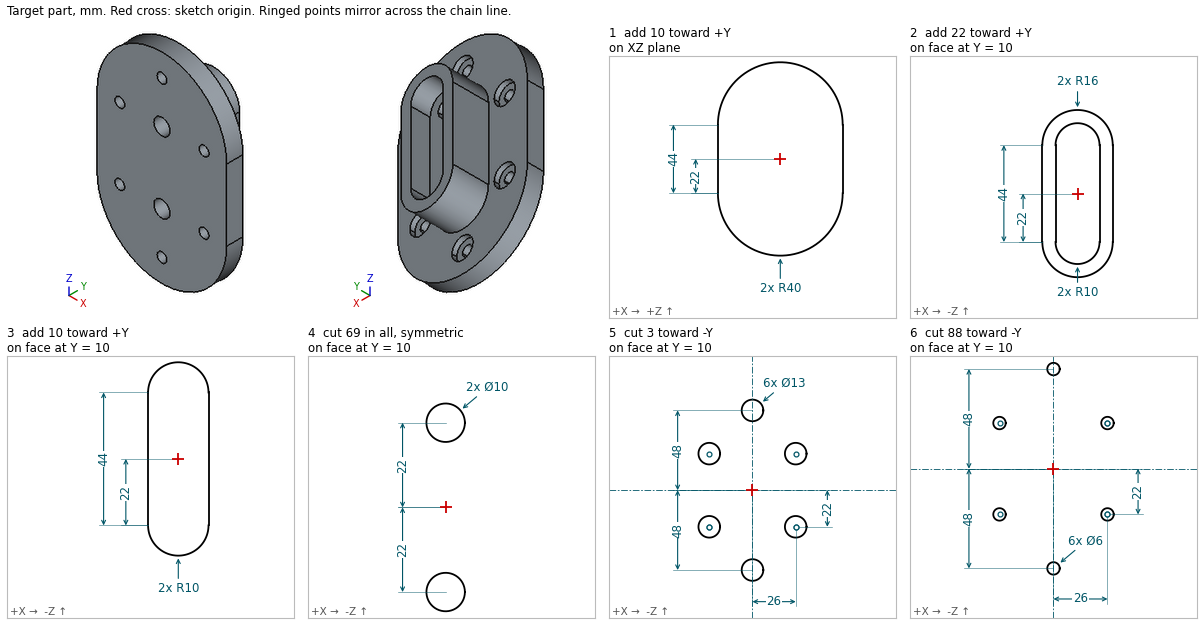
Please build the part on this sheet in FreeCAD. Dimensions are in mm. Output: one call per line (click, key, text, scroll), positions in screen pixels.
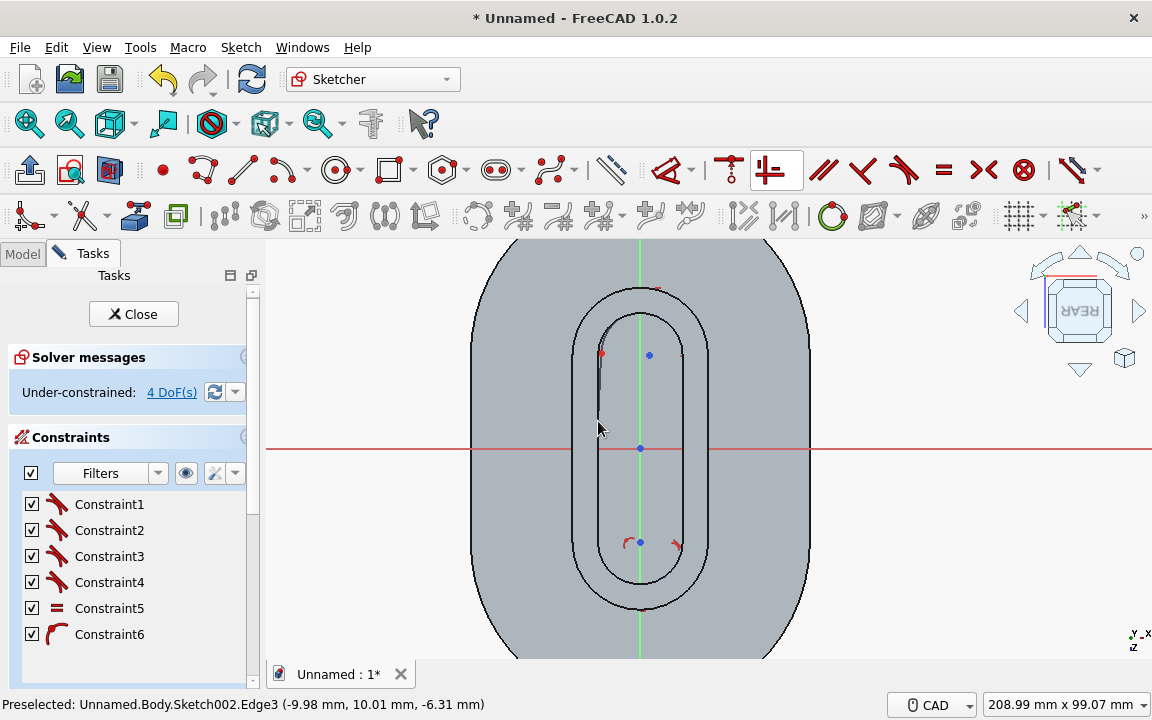
click(595, 485)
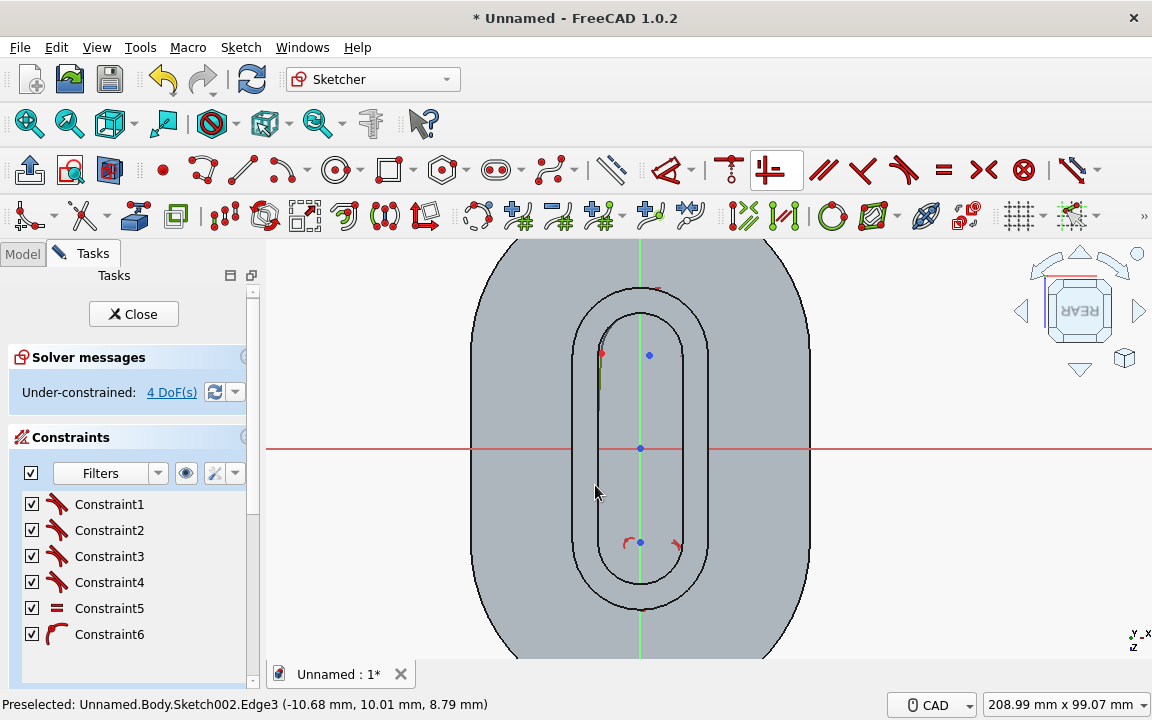
click(798, 170)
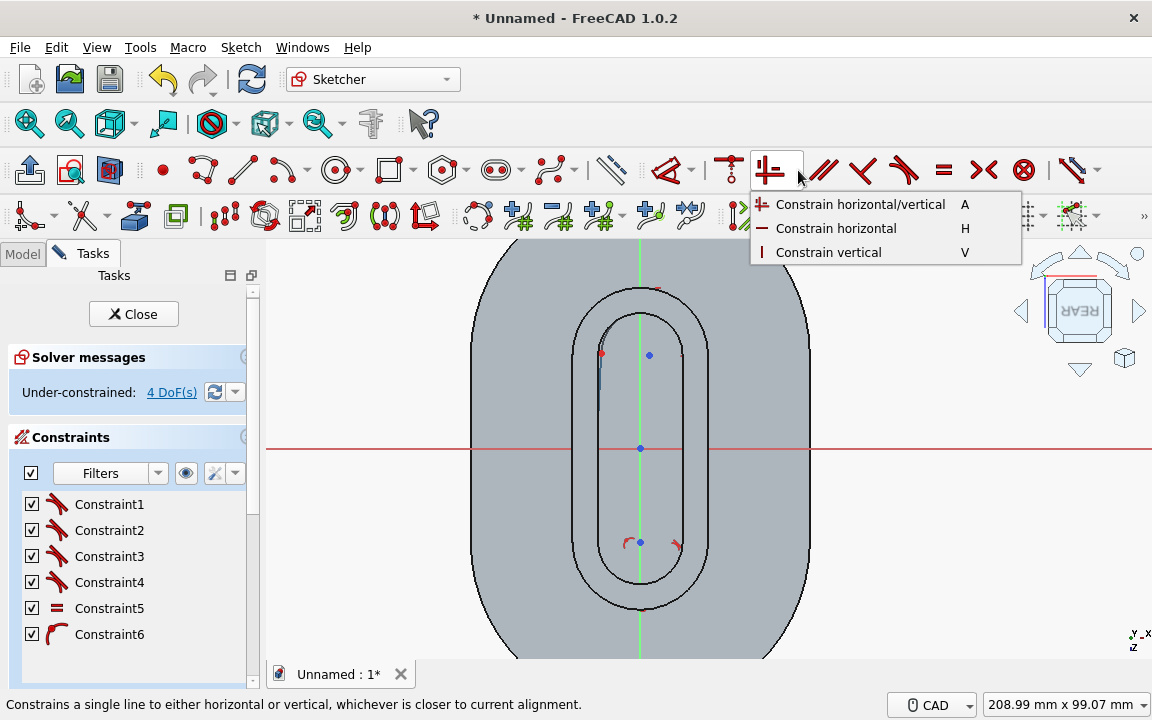
click(886, 252)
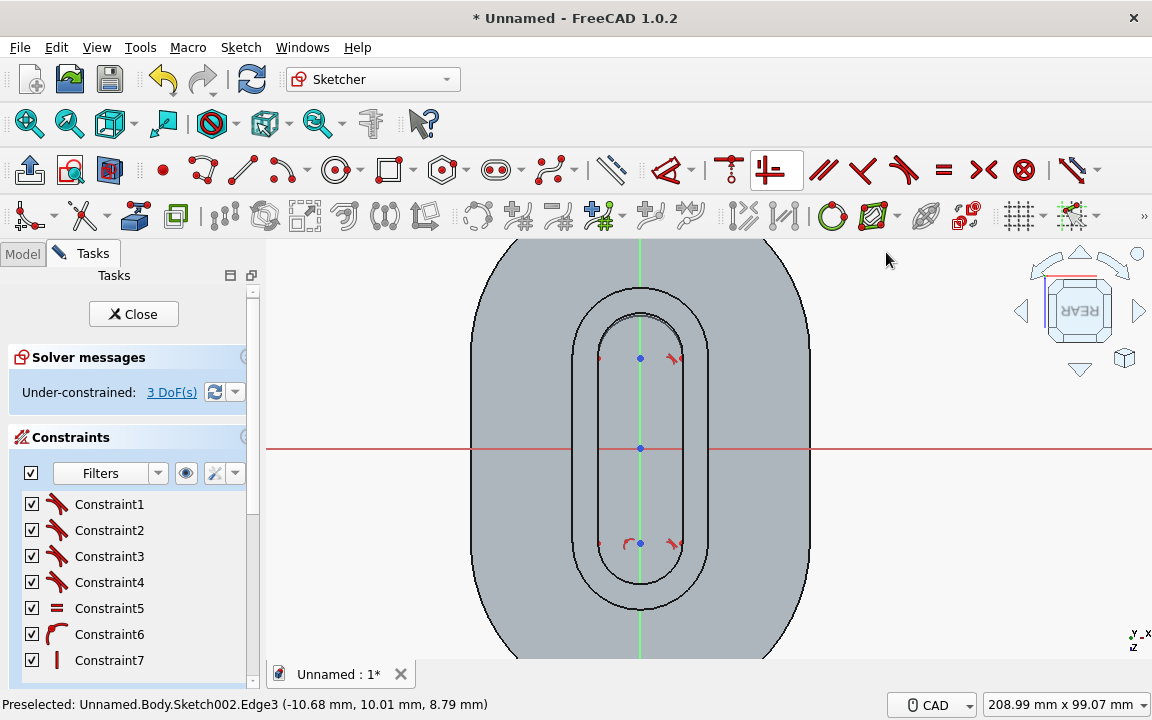
click(666, 170)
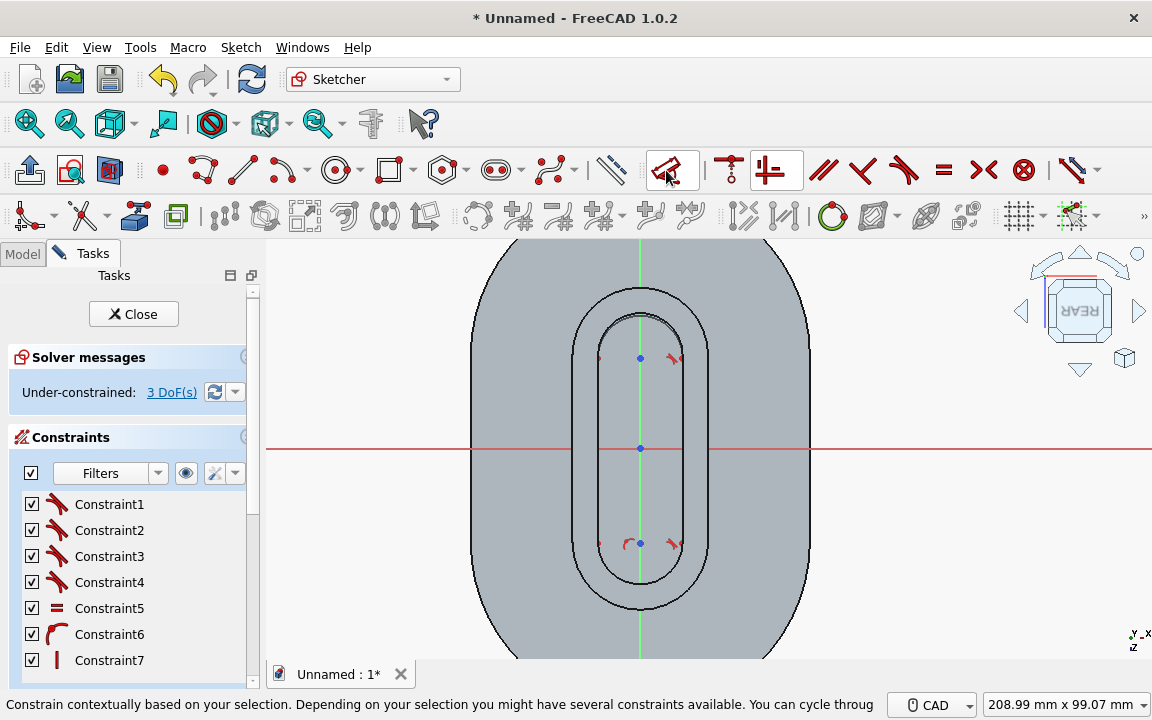
click(615, 577)
click(596, 603)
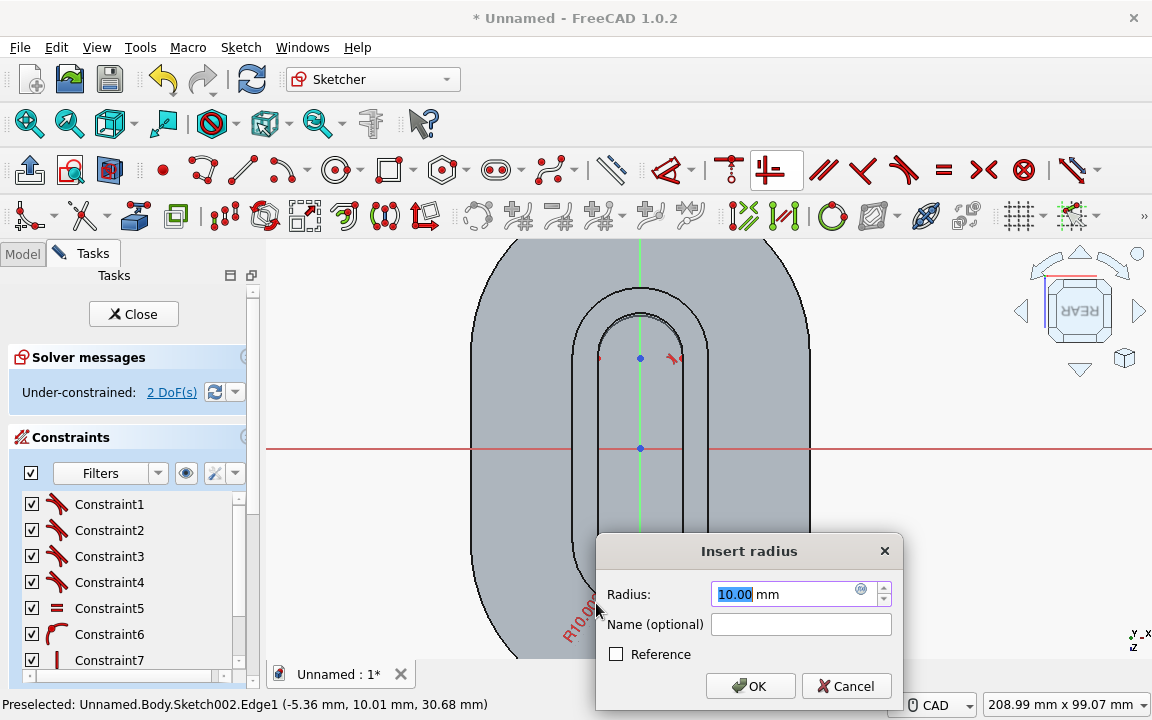
text(10)
key(Return)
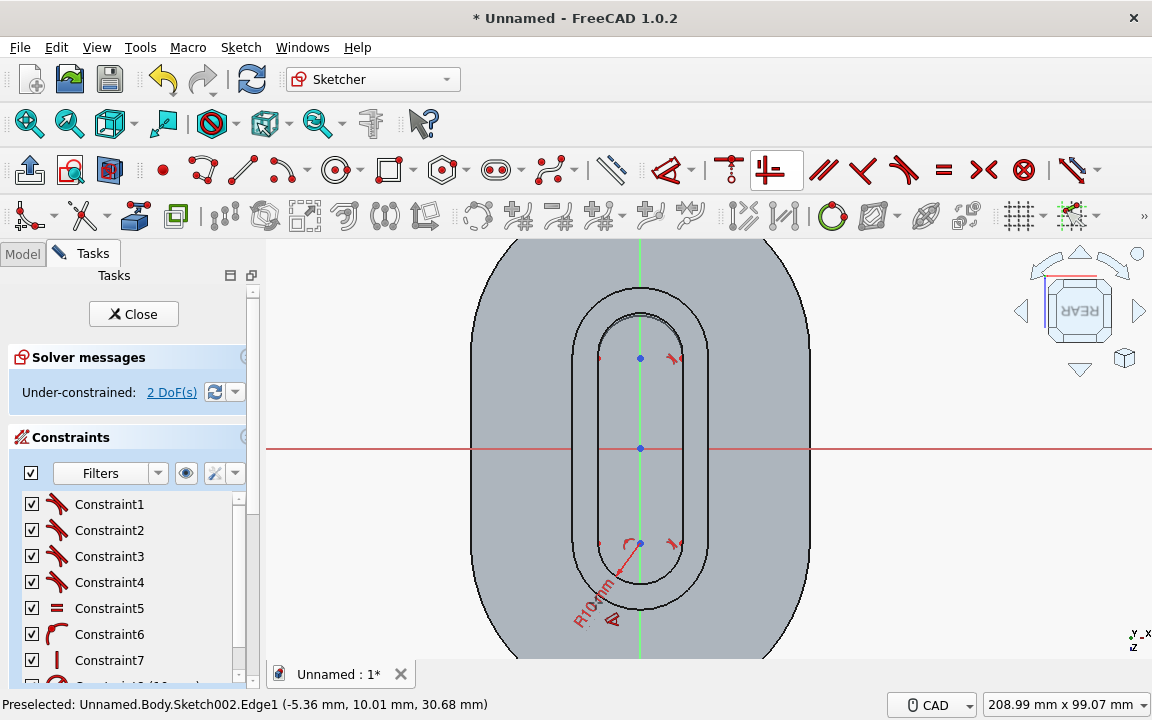
click(598, 488)
click(564, 408)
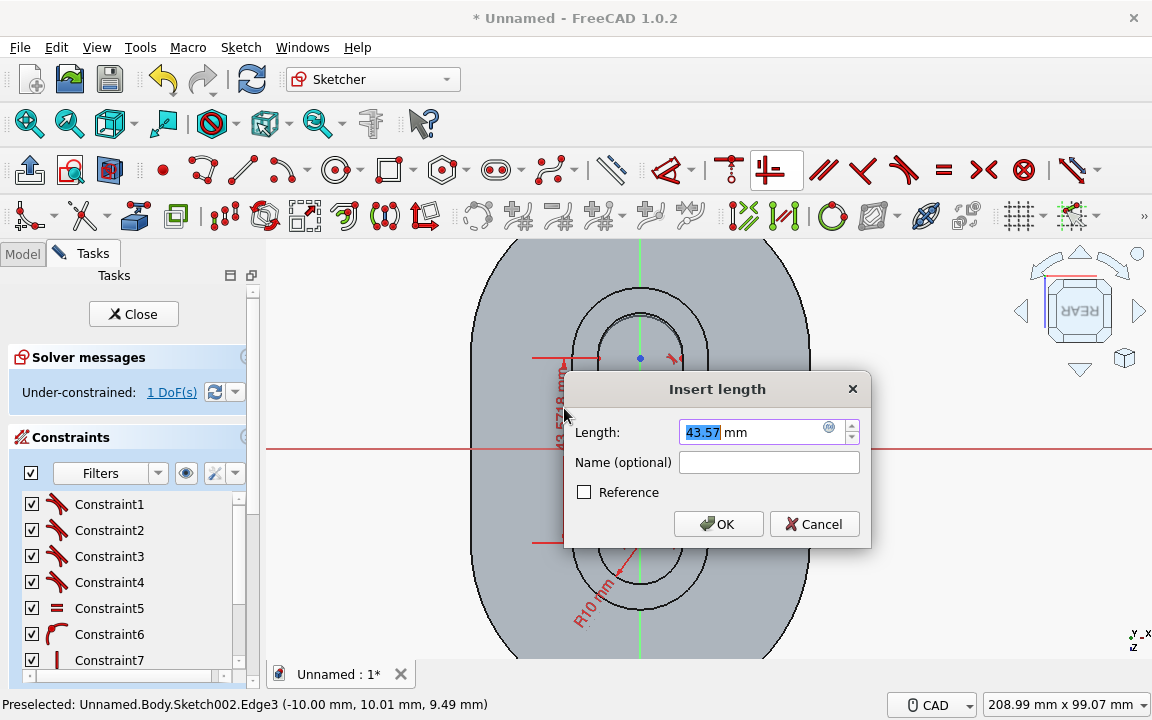
text(44)
key(Return)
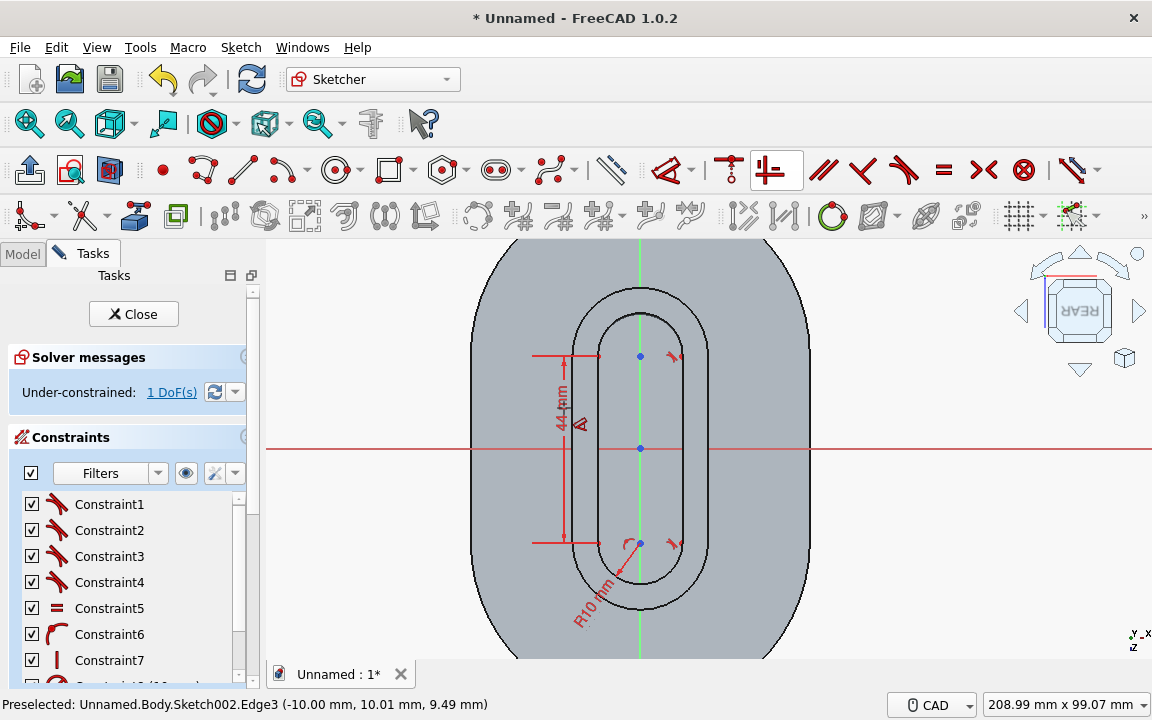
click(598, 543)
click(564, 496)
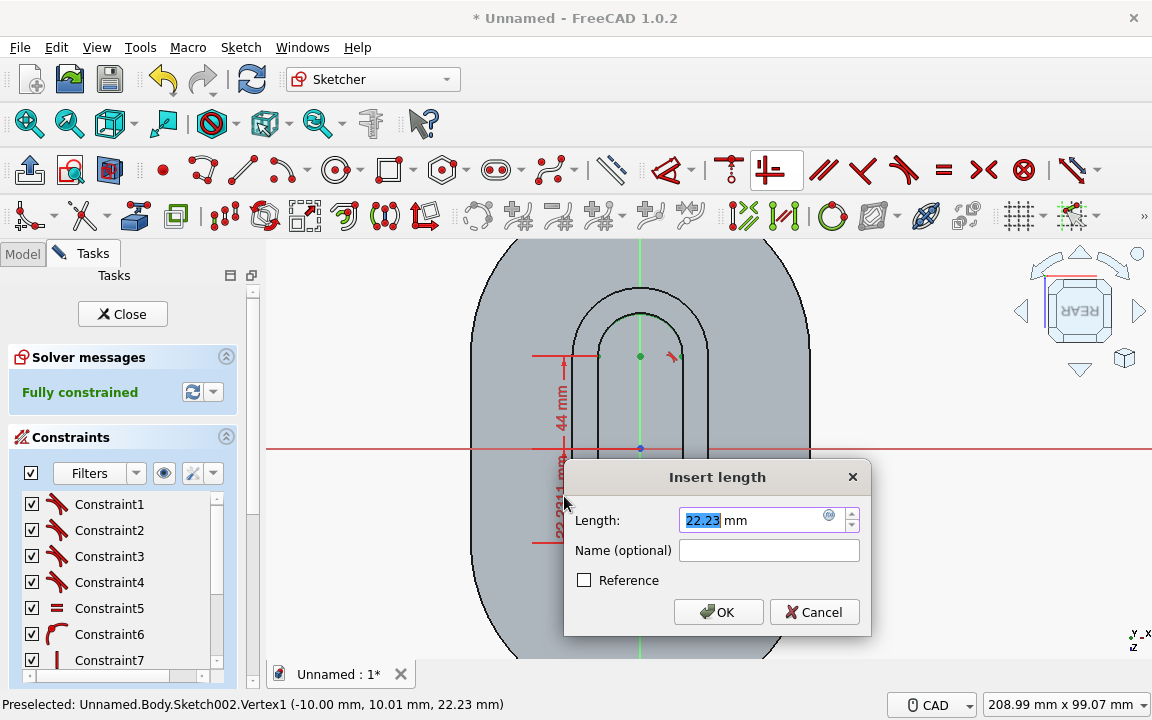
text(22)
key(Return)
key(Escape)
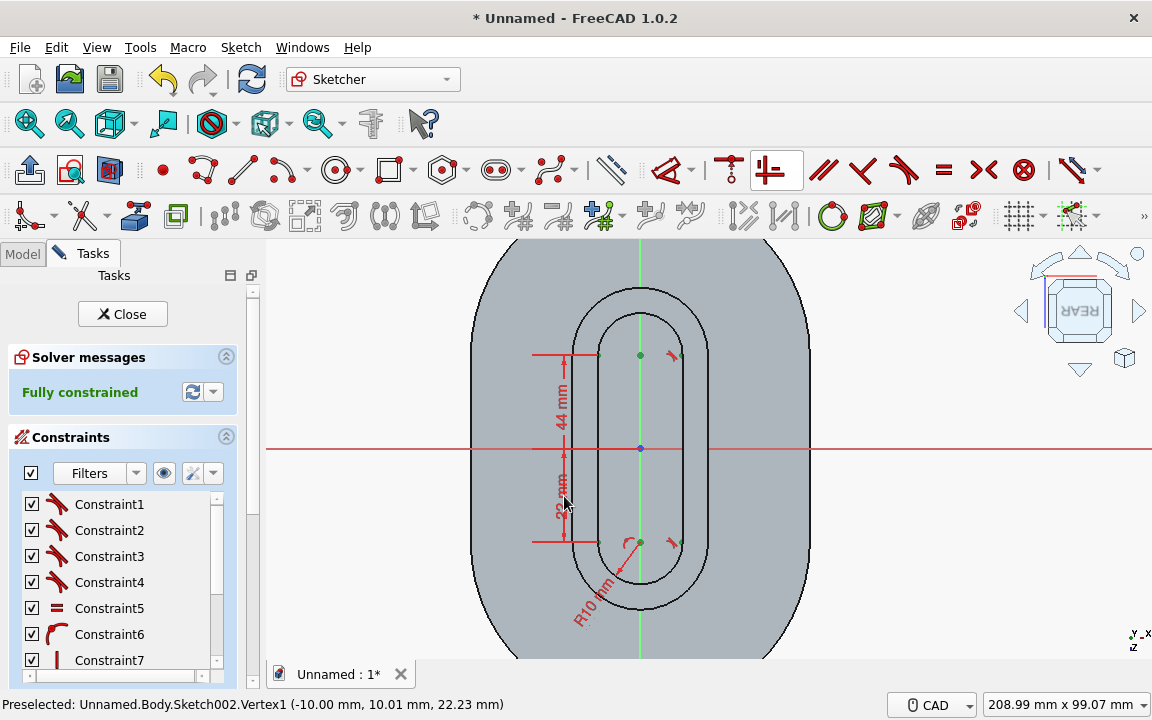
click(123, 314)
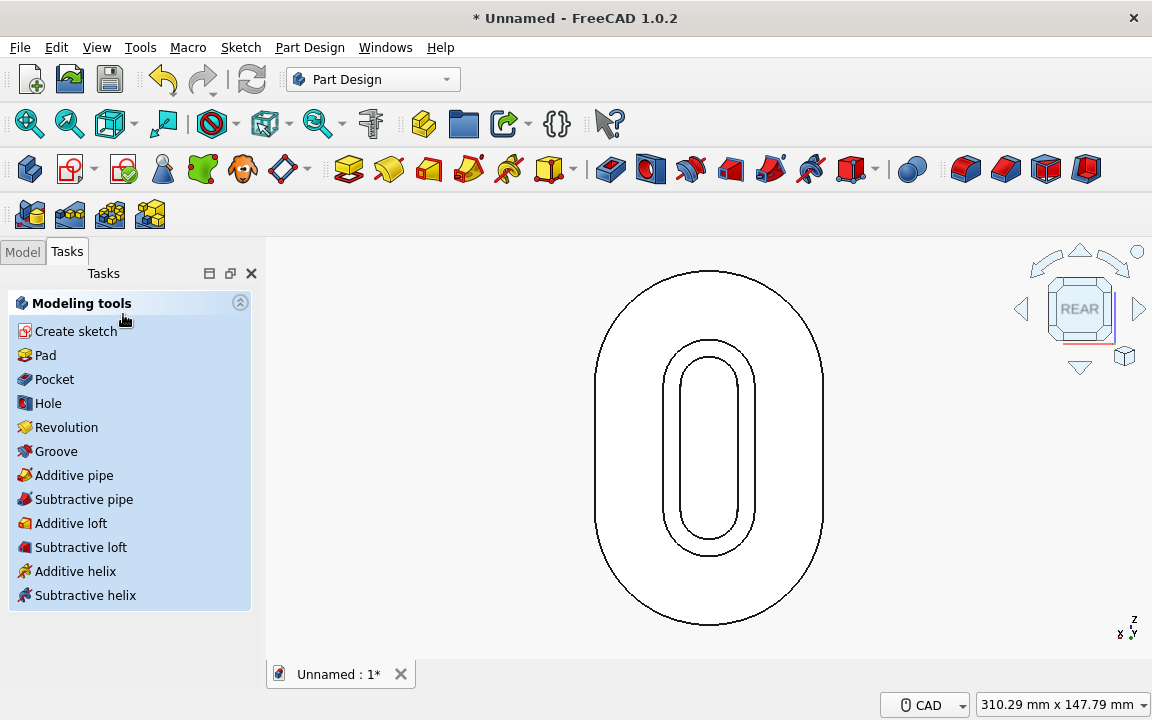
click(350, 170)